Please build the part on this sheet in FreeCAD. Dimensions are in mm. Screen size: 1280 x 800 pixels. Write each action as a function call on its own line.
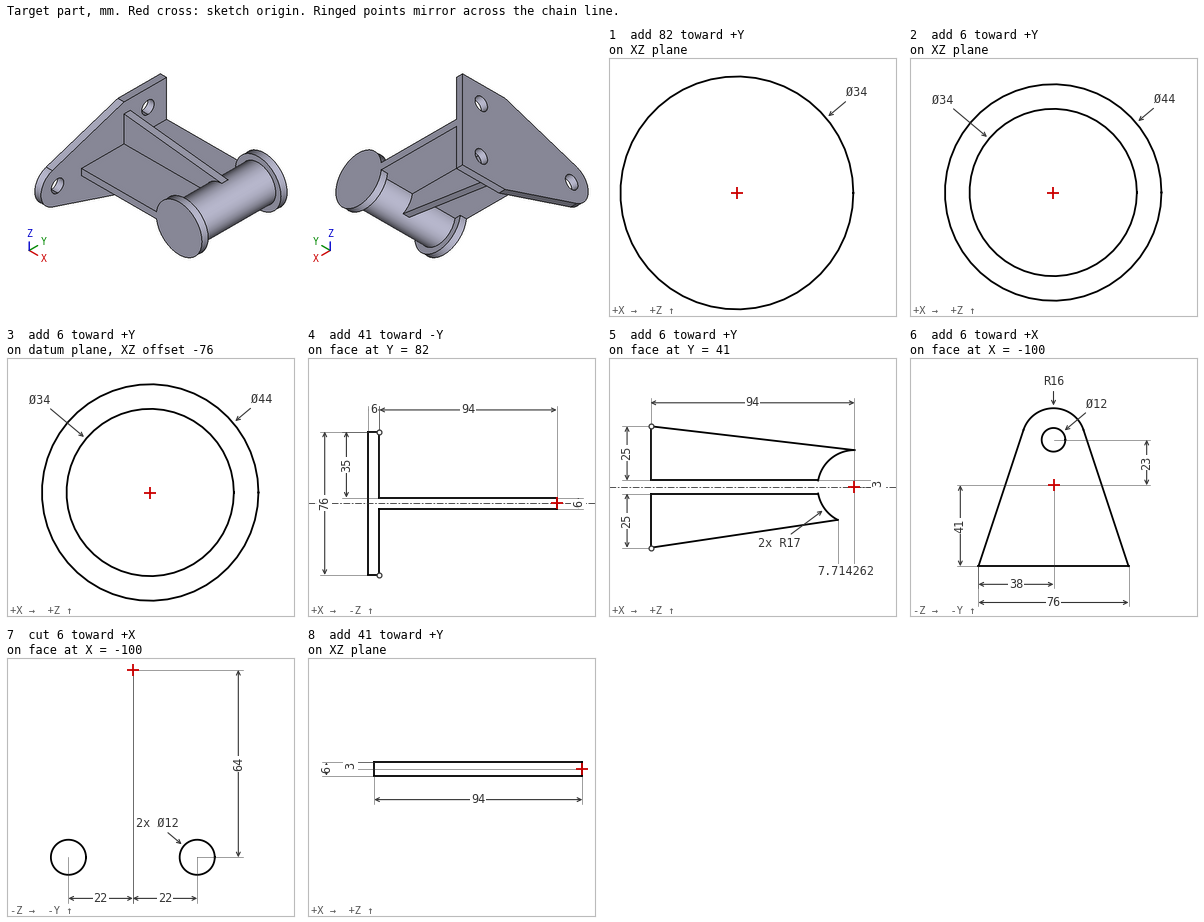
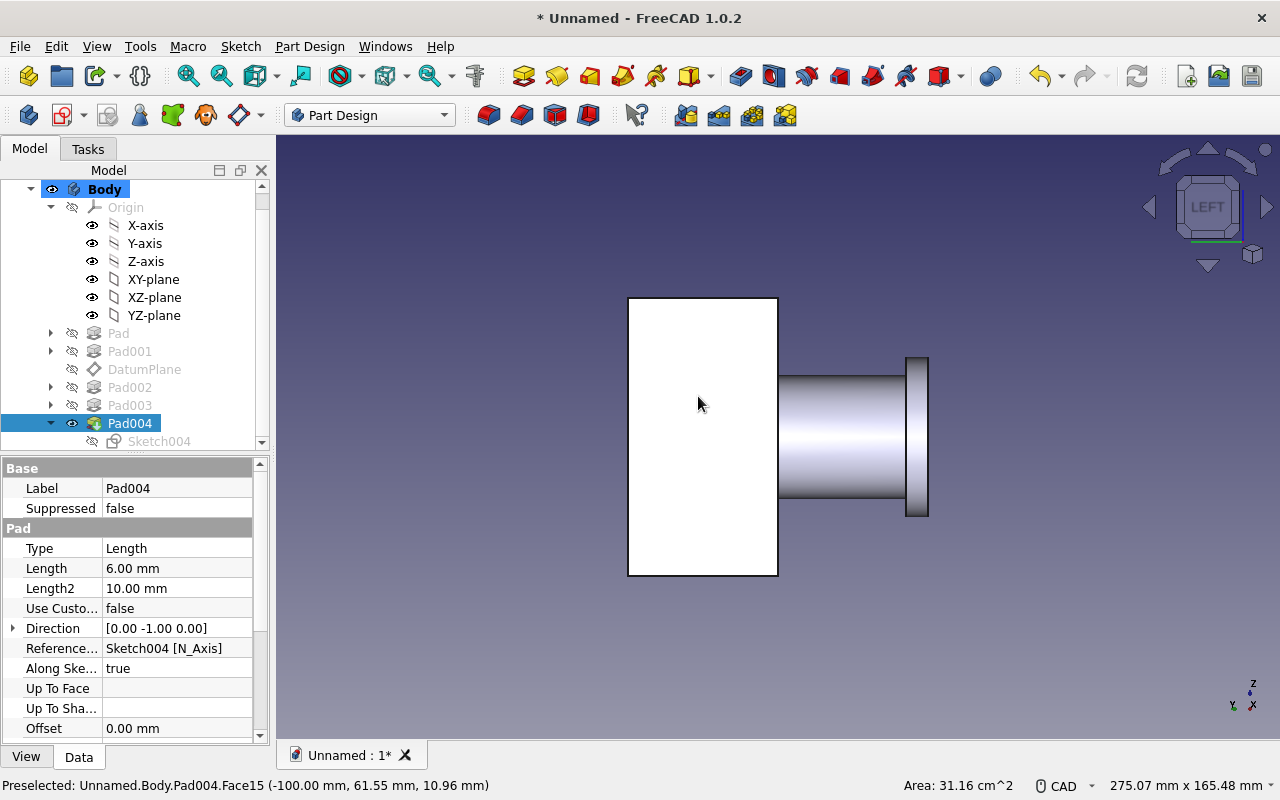
click(62, 116)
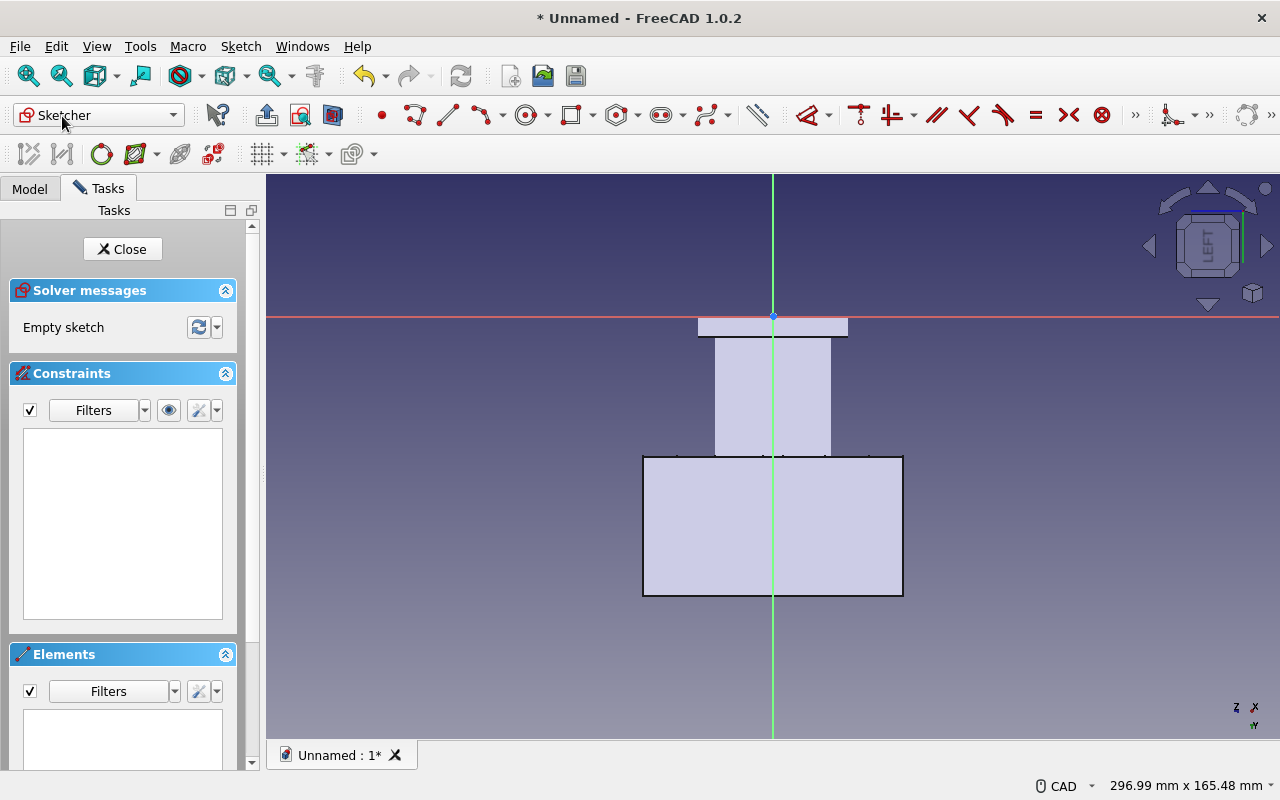
scroll(395, 711, down, 1)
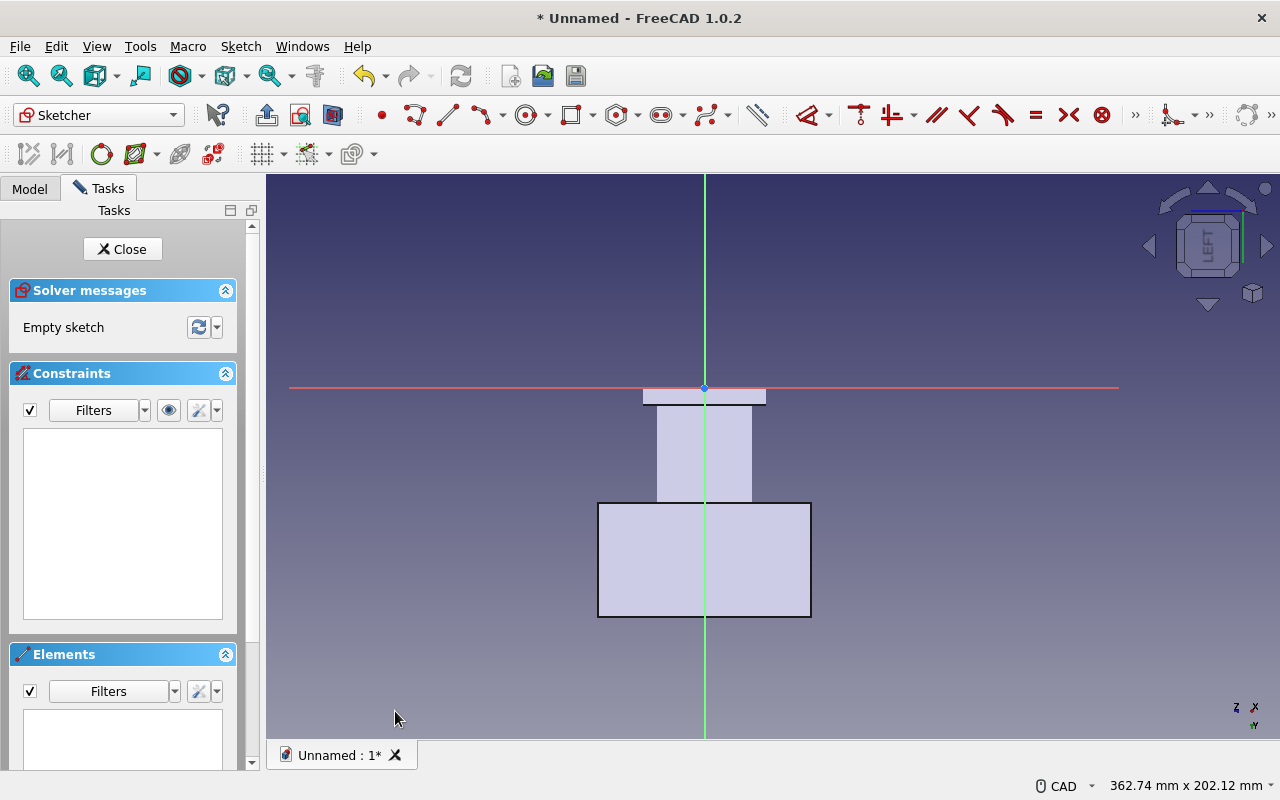
scroll(705, 258, up, 2)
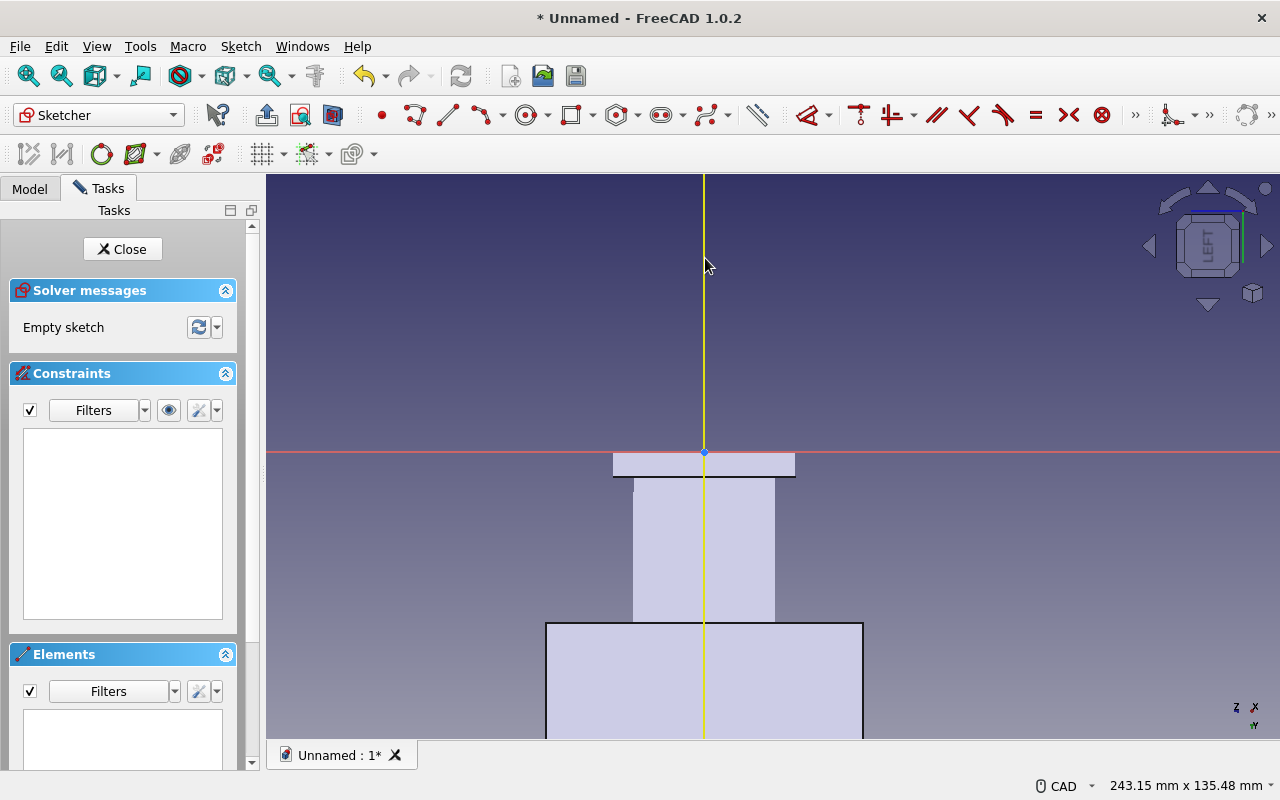
click(415, 116)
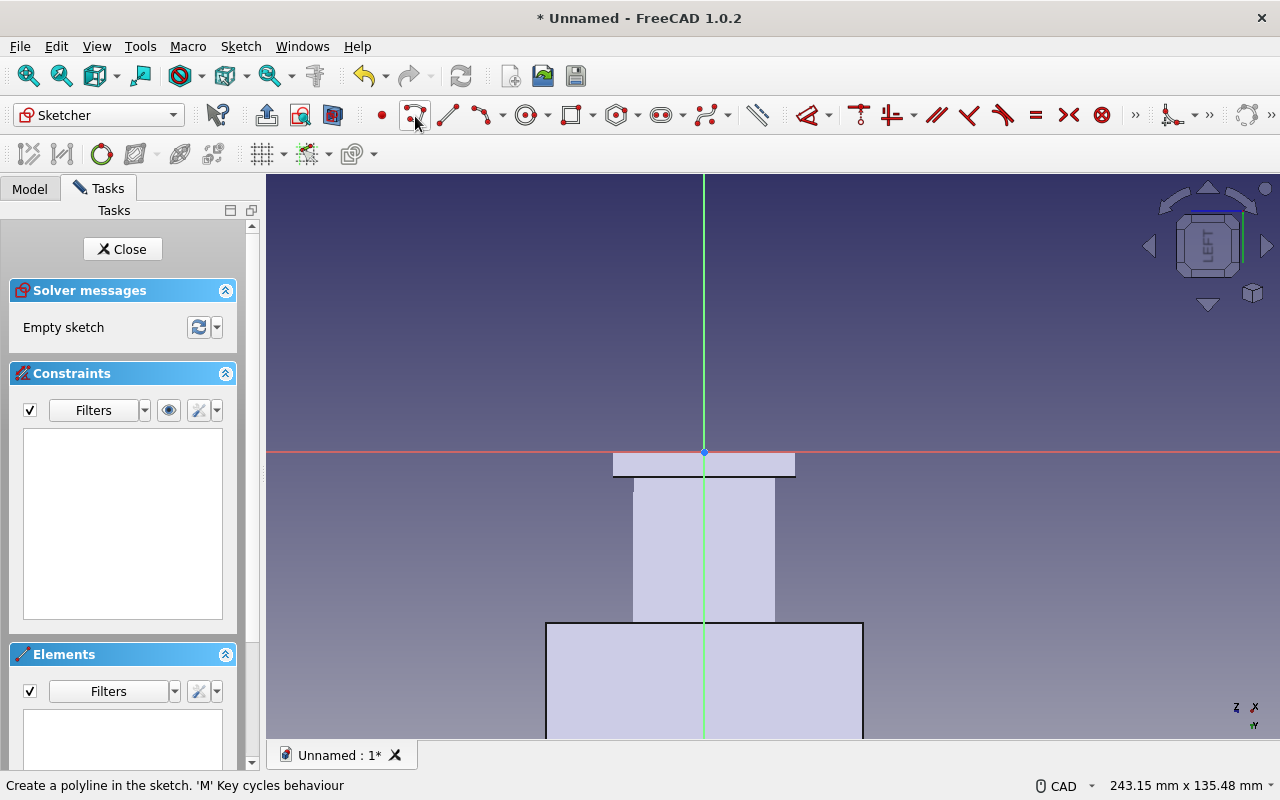
click(641, 335)
click(546, 623)
click(863, 623)
click(767, 335)
right_click(767, 335)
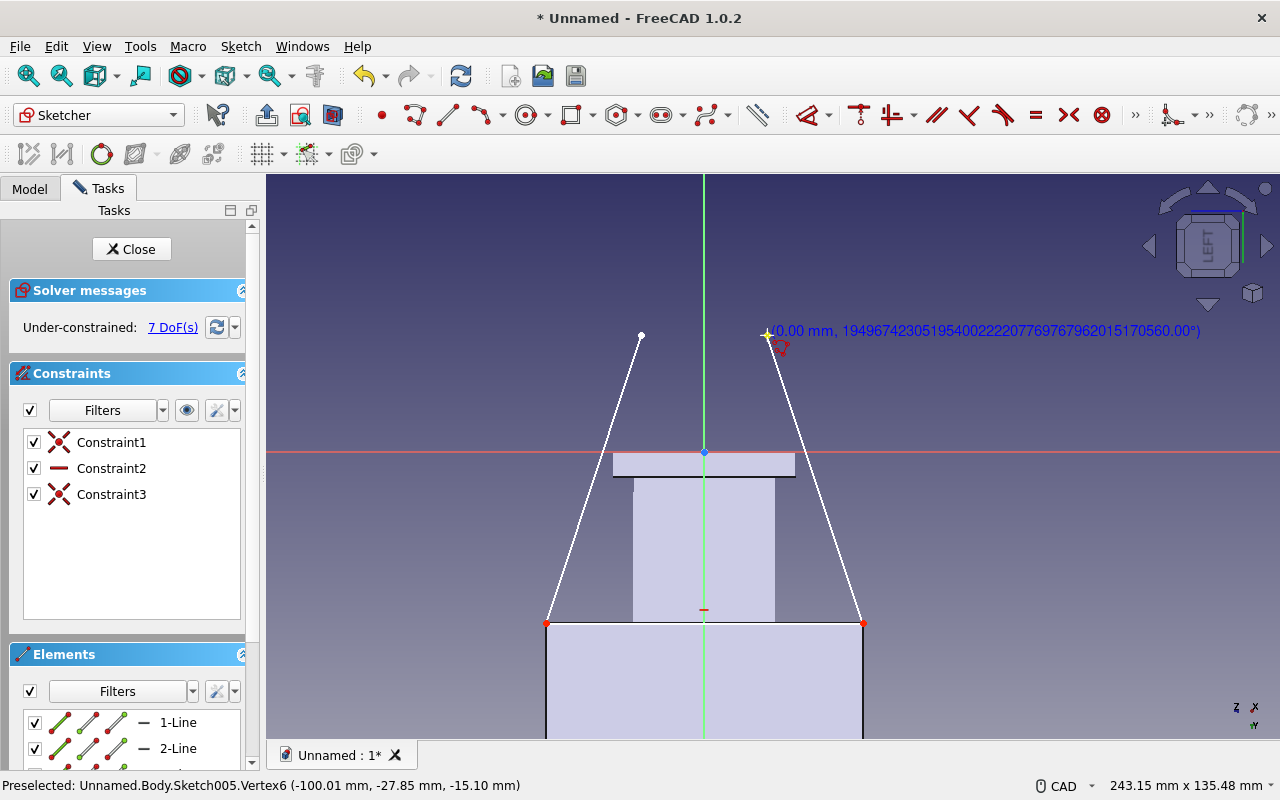
click(480, 116)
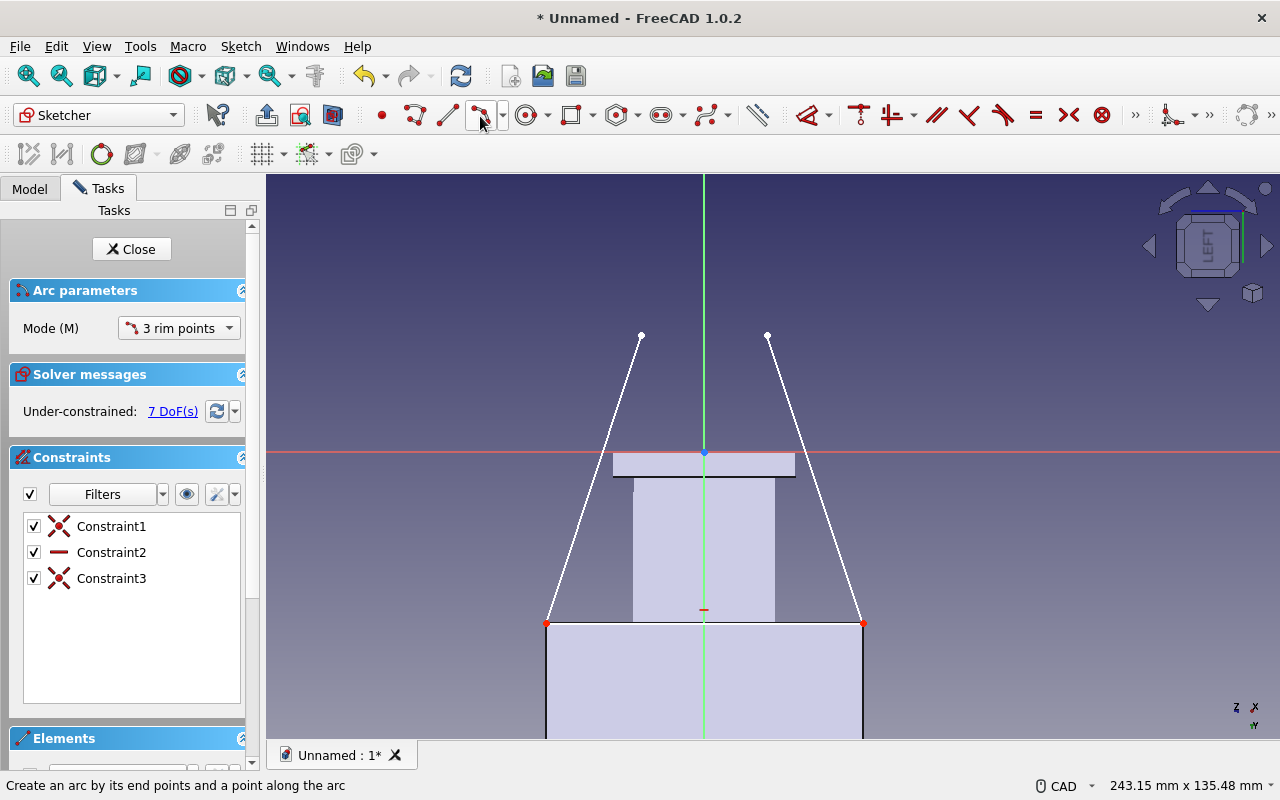
click(767, 336)
click(641, 336)
click(721, 292)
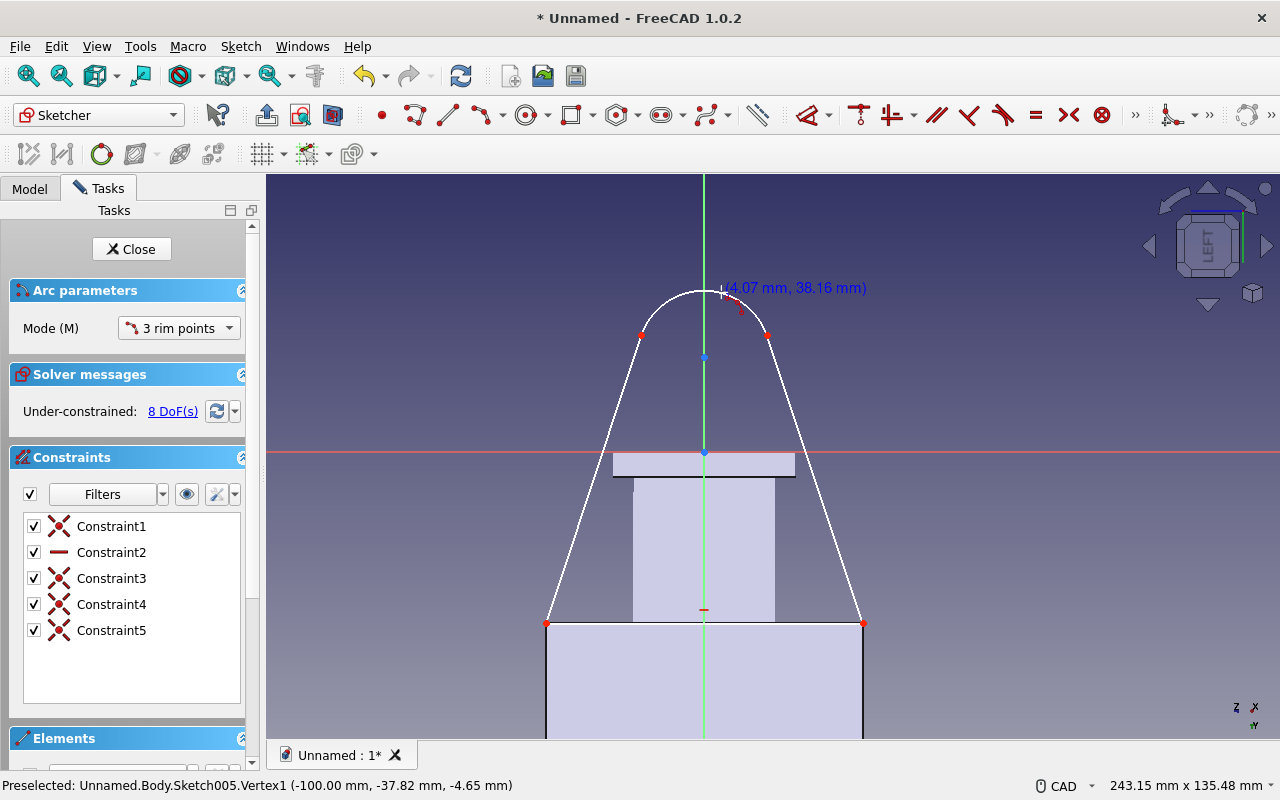
click(526, 116)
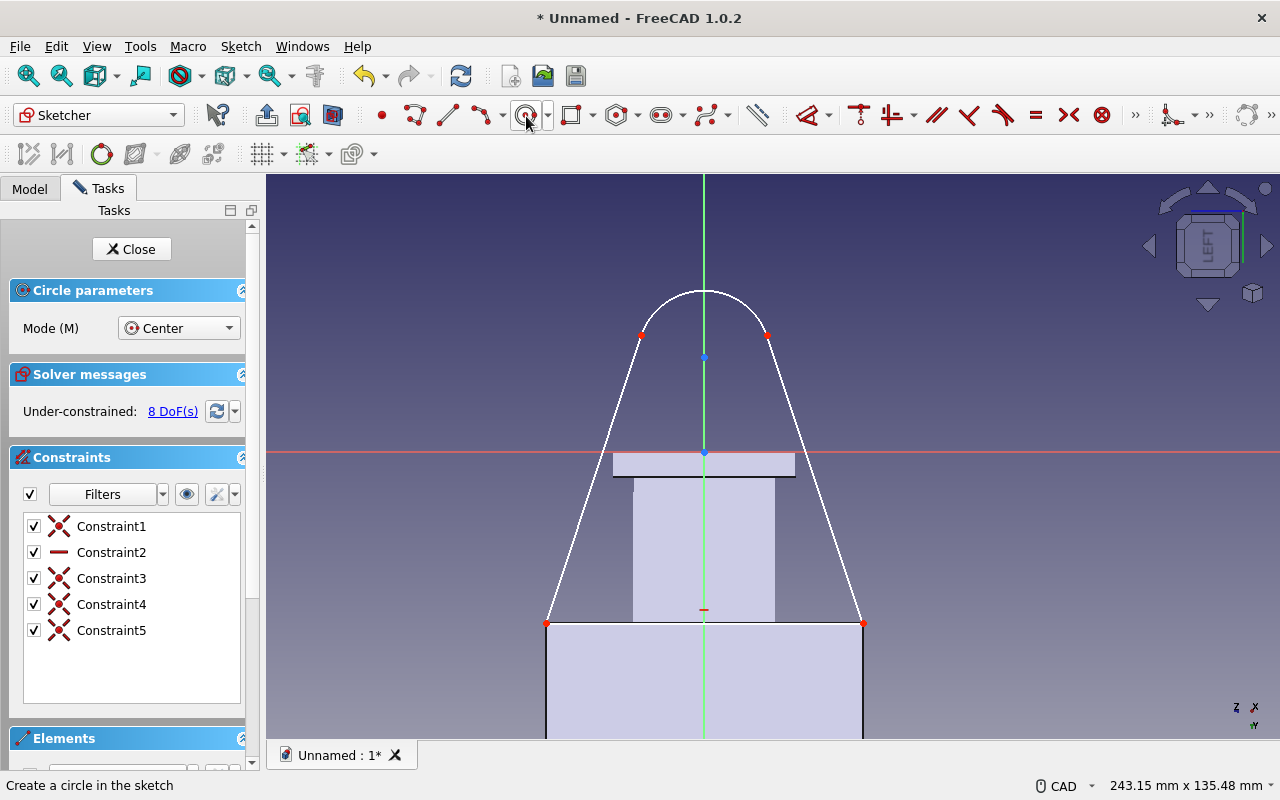
click(704, 356)
click(722, 339)
key(Escape)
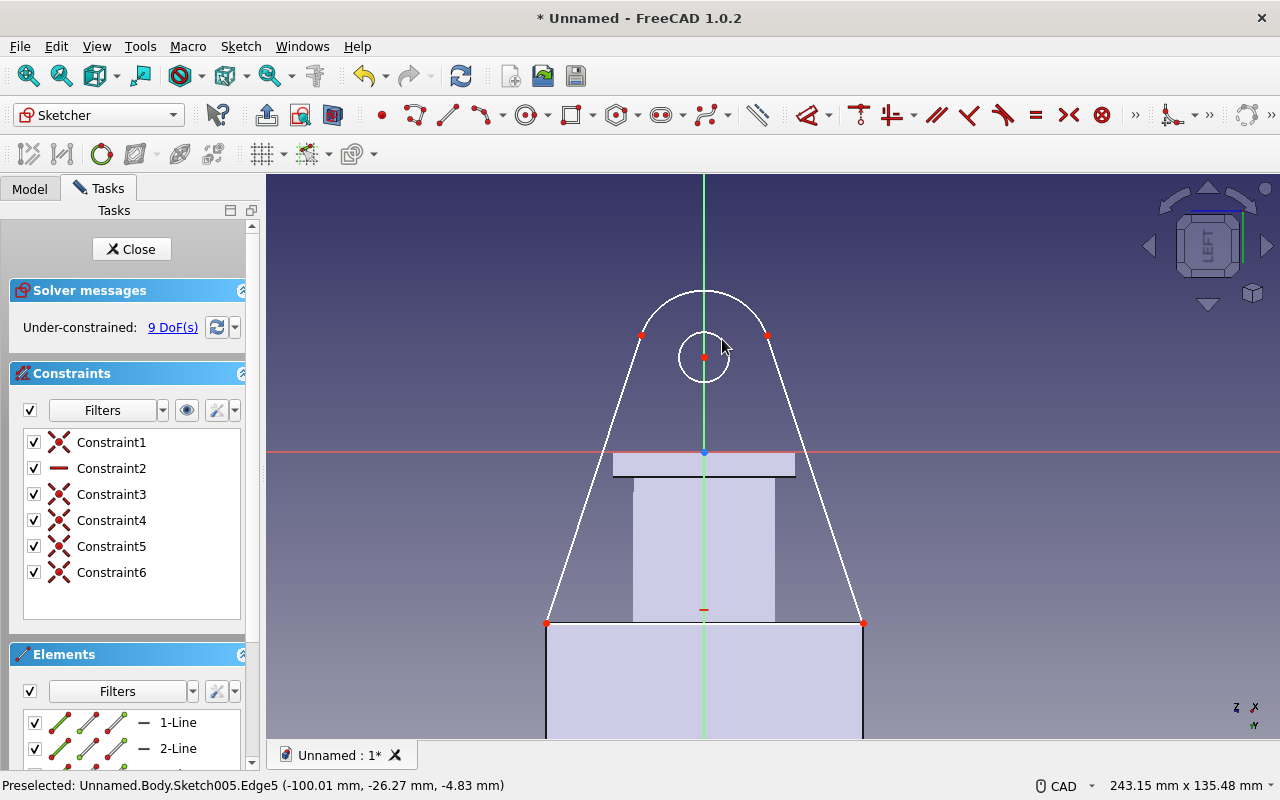
click(613, 422)